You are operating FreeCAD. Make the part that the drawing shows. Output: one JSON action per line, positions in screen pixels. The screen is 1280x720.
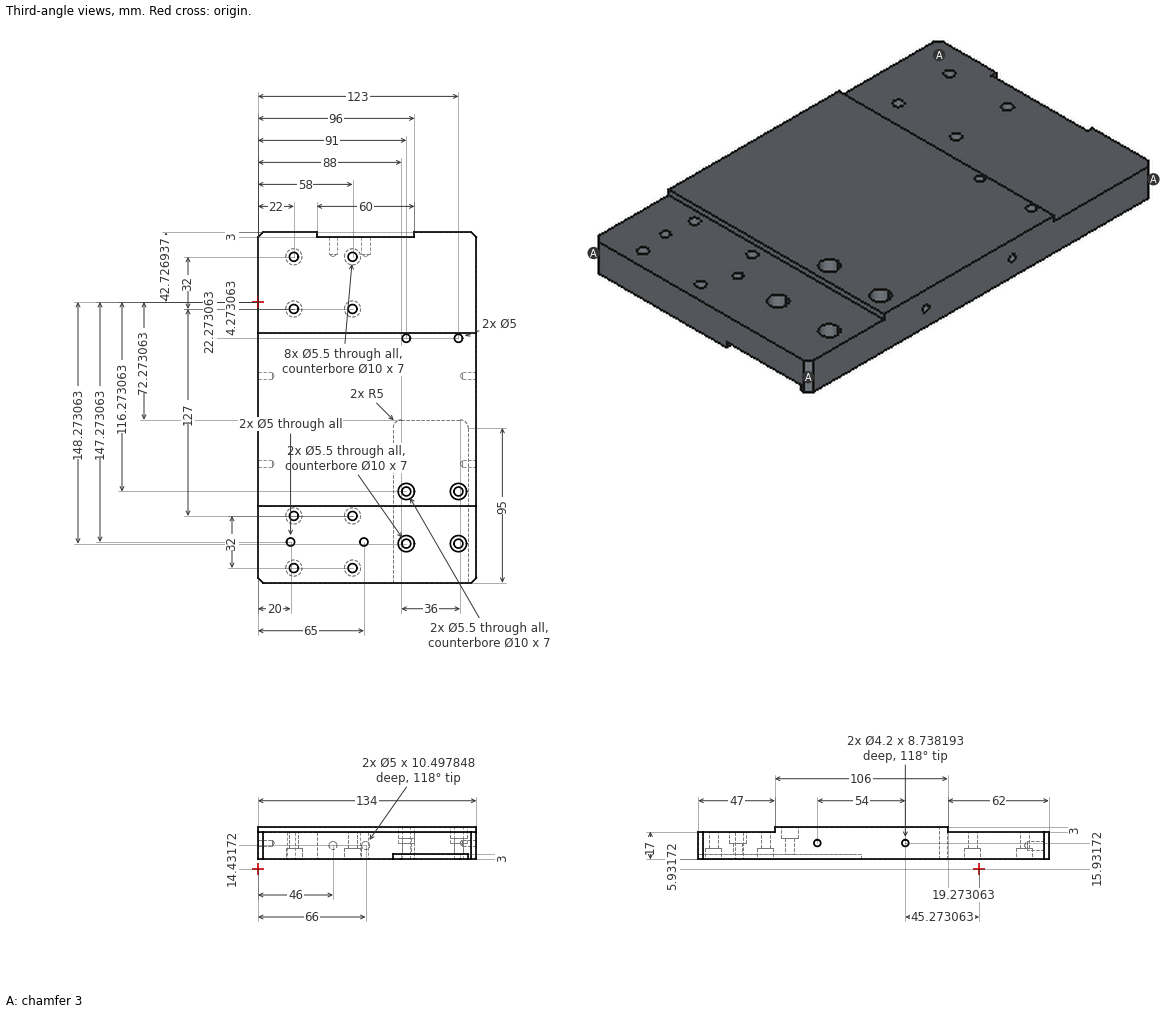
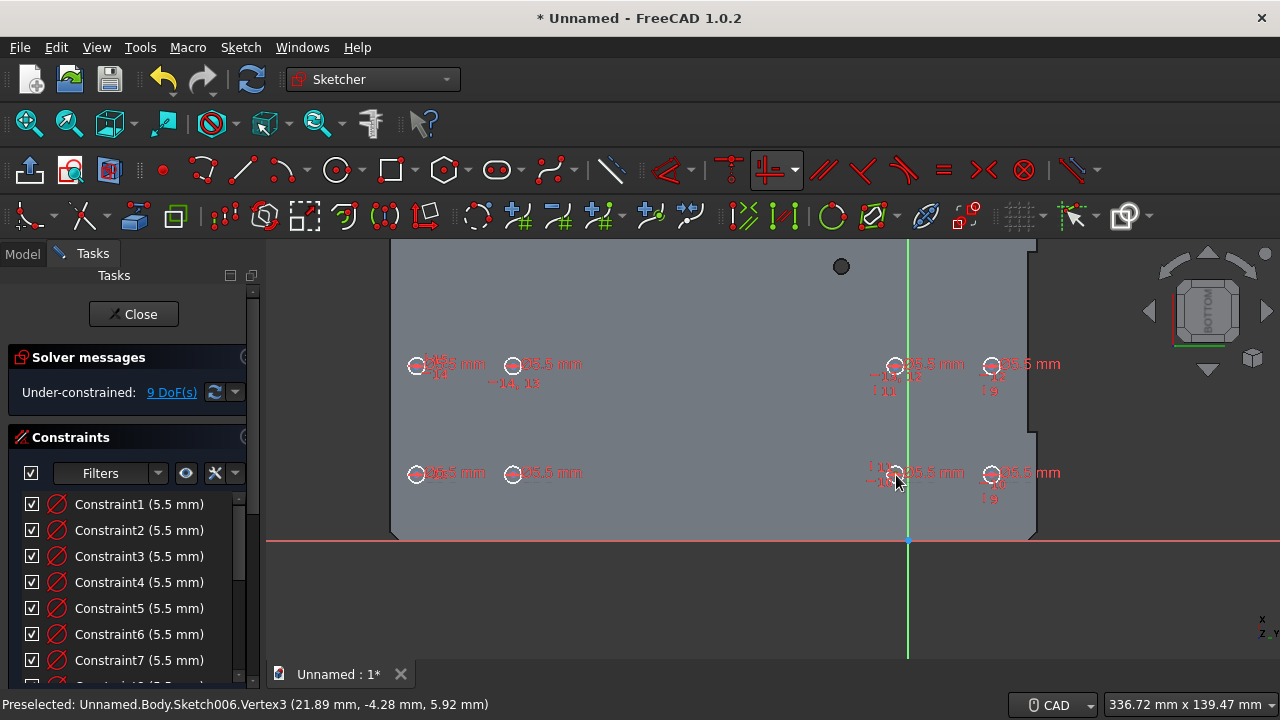
{"action": "left_click", "coordinate": [417, 475]}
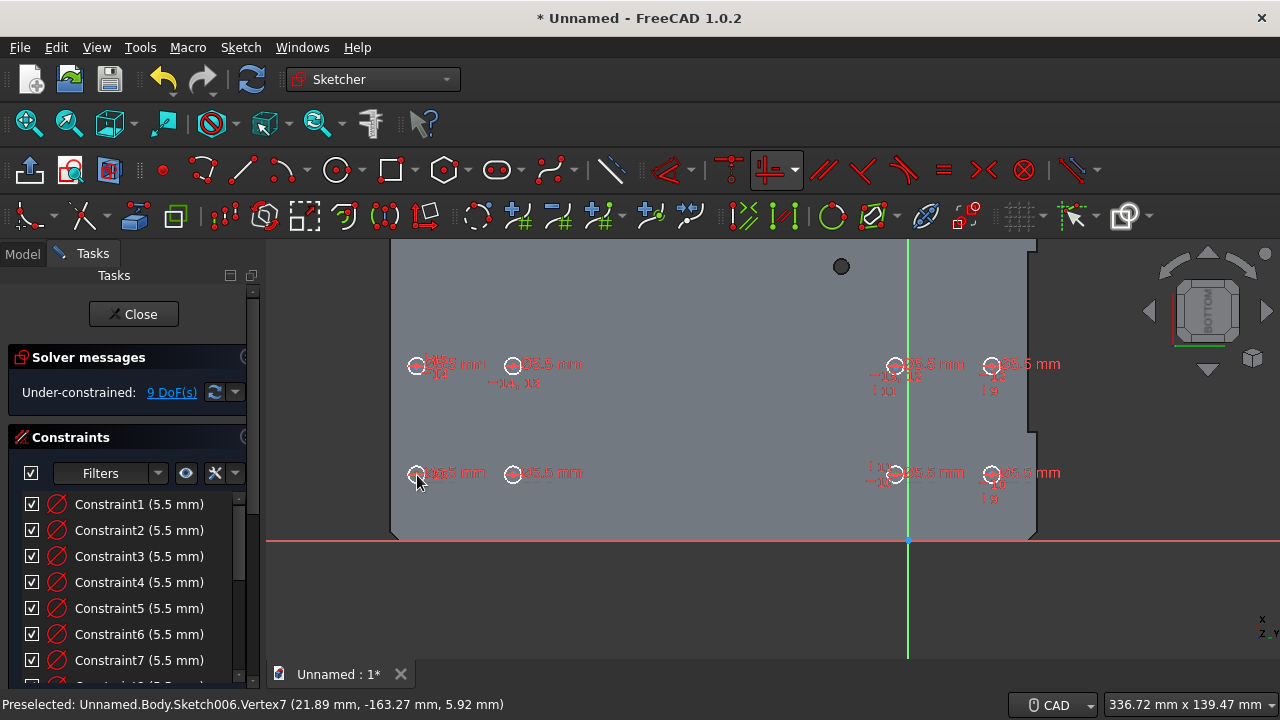
{"action": "key", "text": "h"}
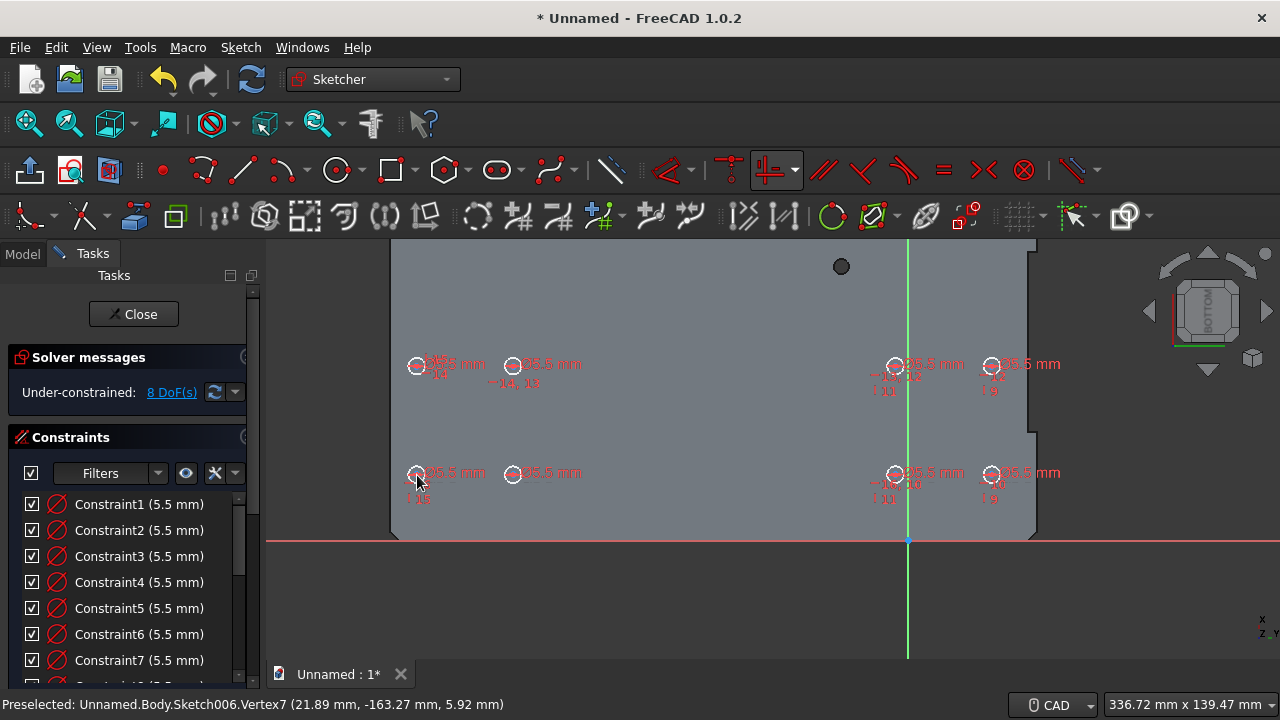
{"action": "left_click", "coordinate": [513, 366]}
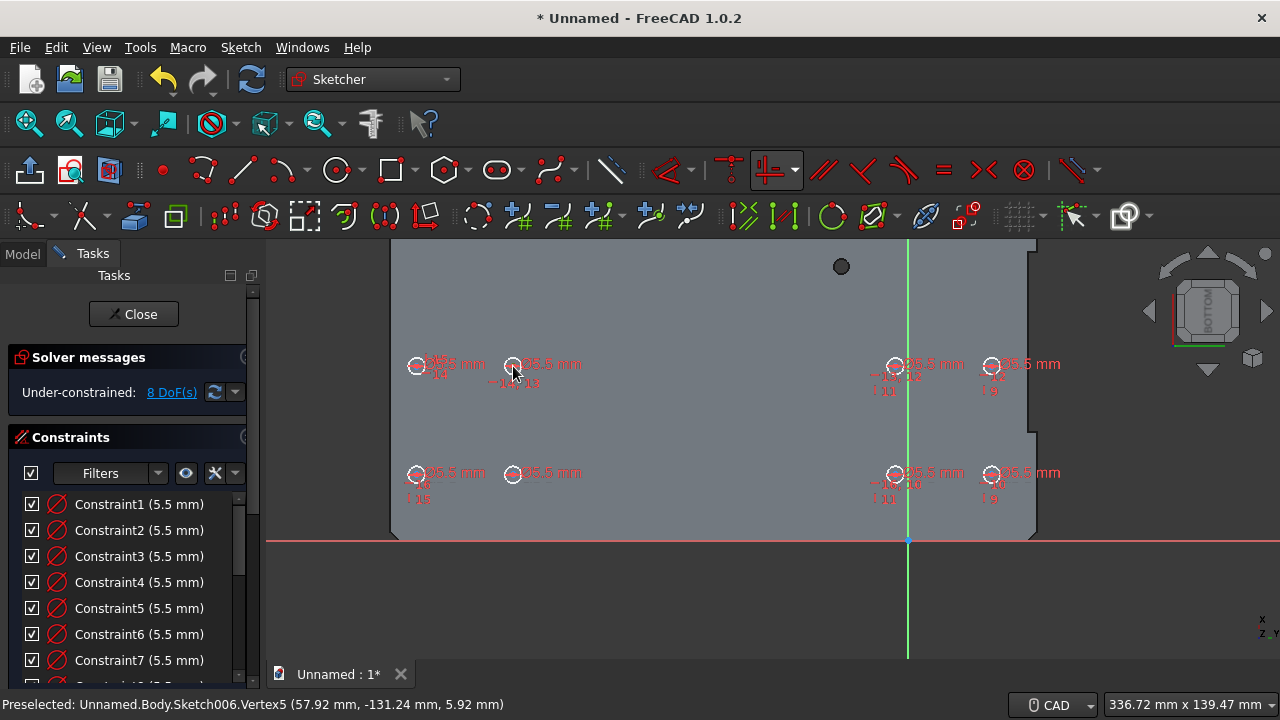
{"action": "left_click", "coordinate": [513, 475]}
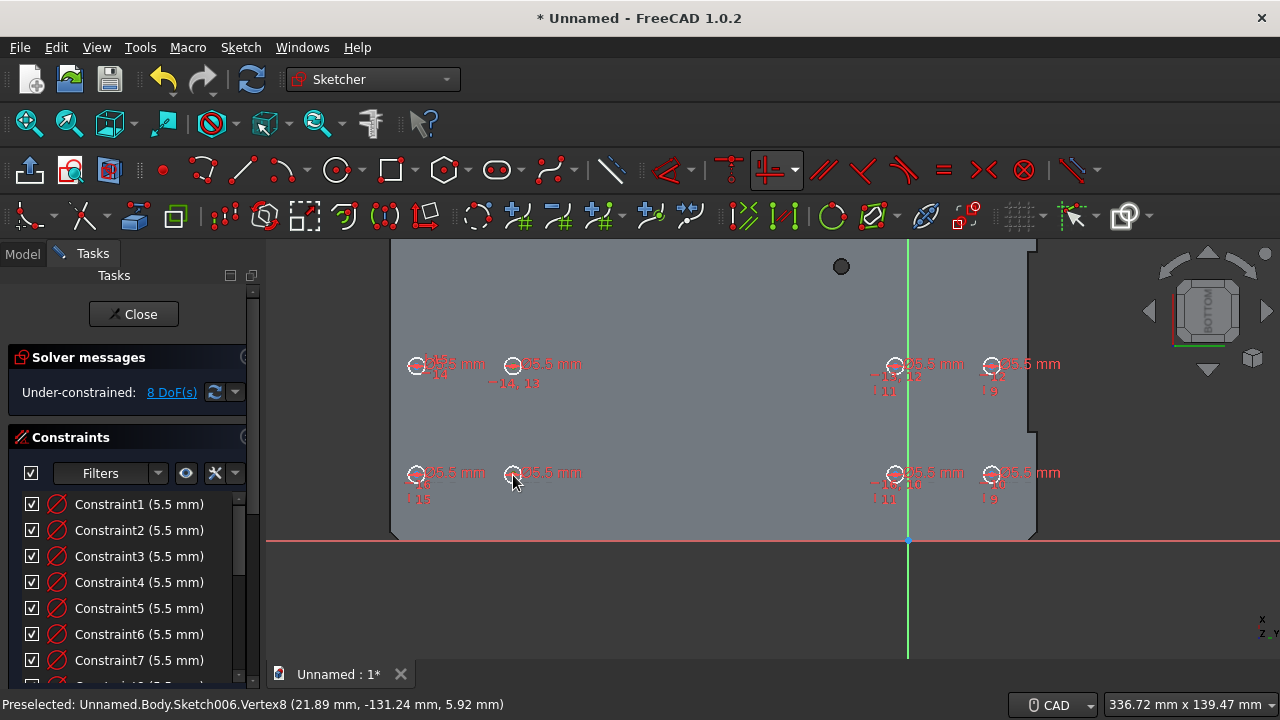
{"action": "left_click", "coordinate": [798, 170]}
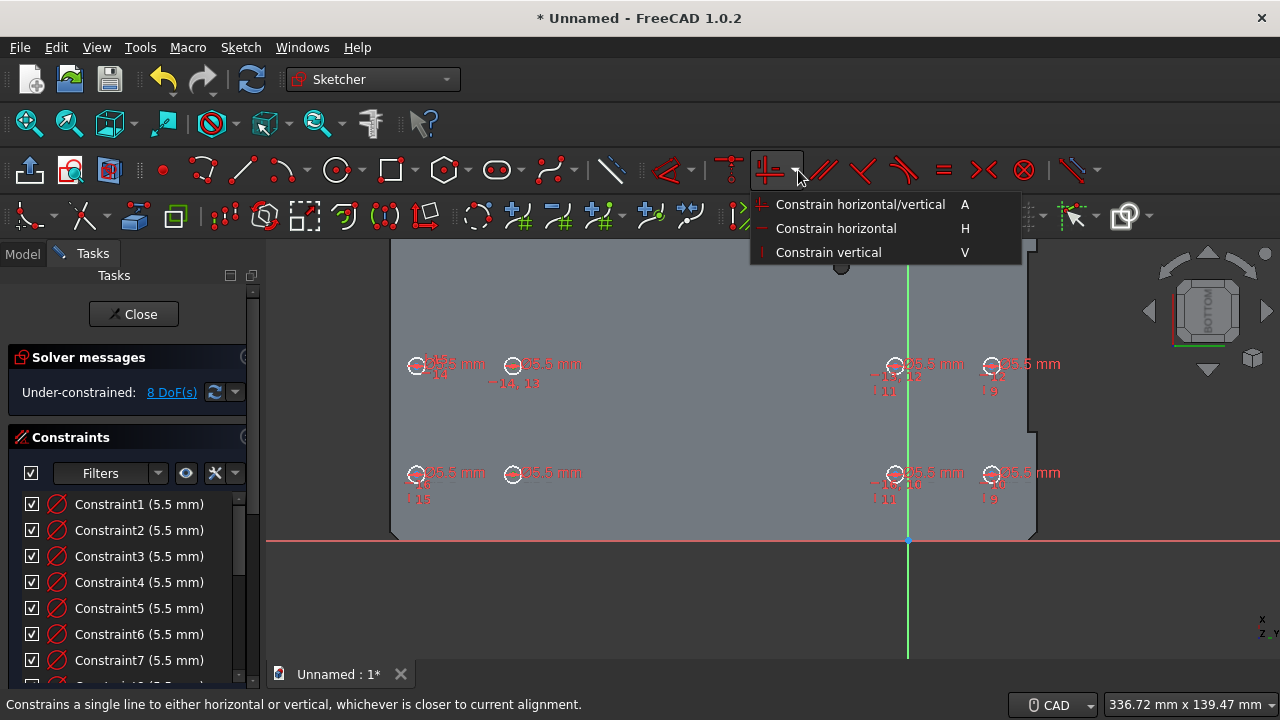
{"action": "left_click", "coordinate": [886, 252]}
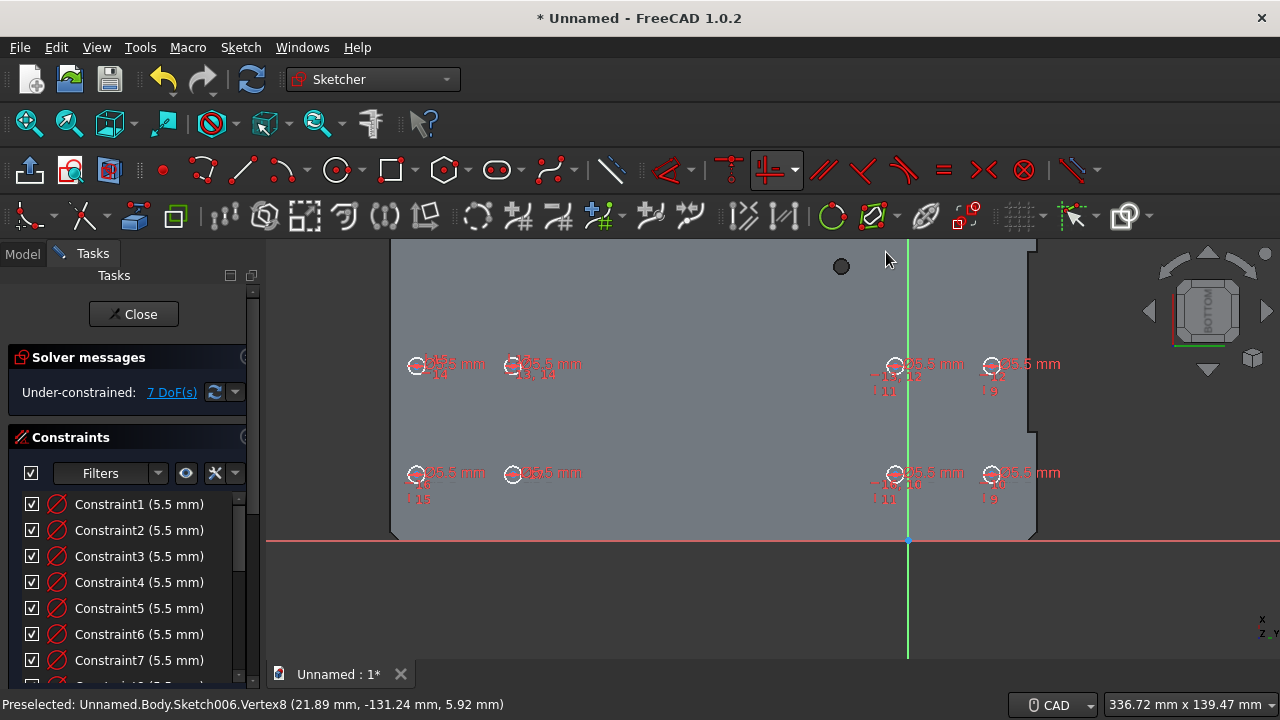
{"action": "left_click", "coordinate": [417, 475]}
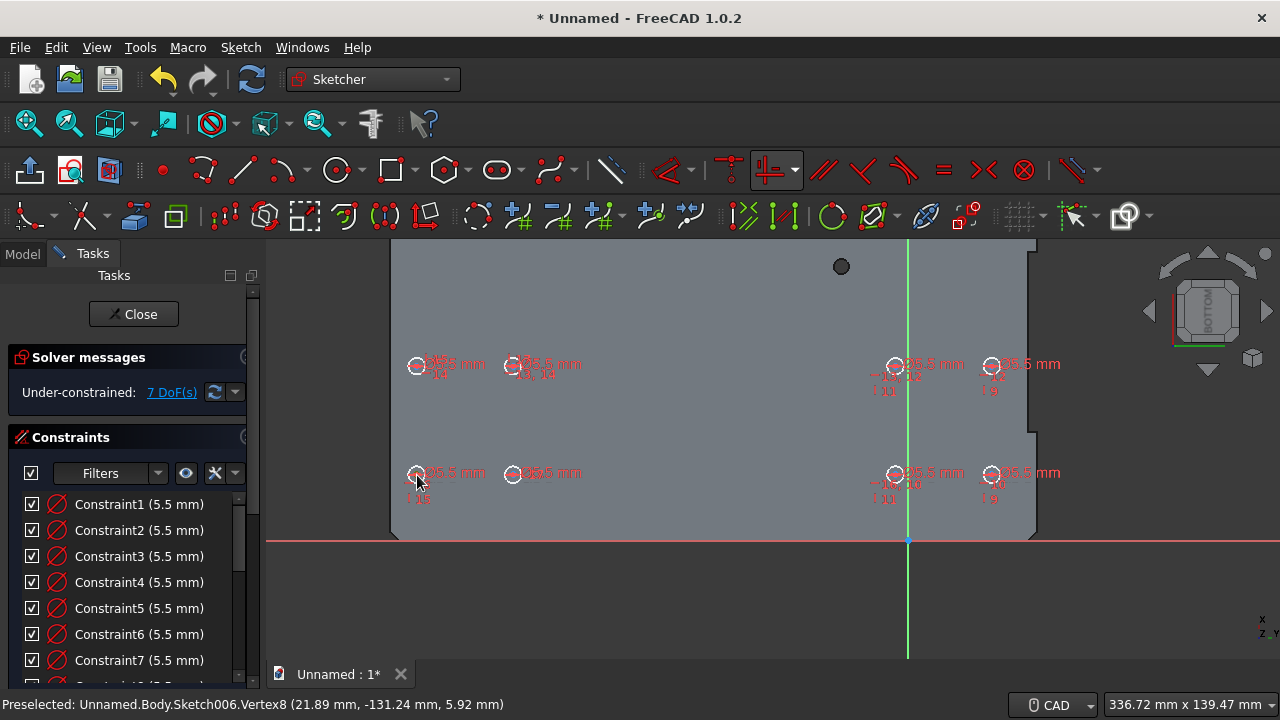
{"action": "left_click", "coordinate": [513, 475]}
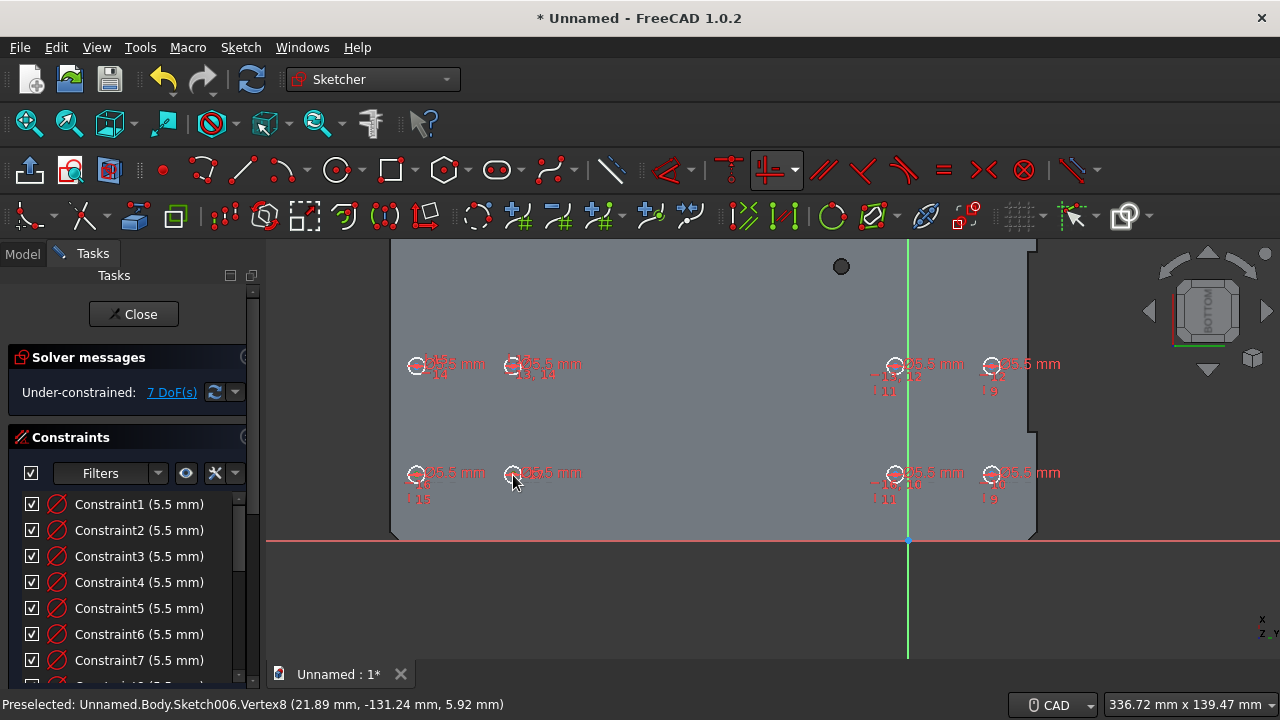
{"action": "left_click", "coordinate": [798, 170]}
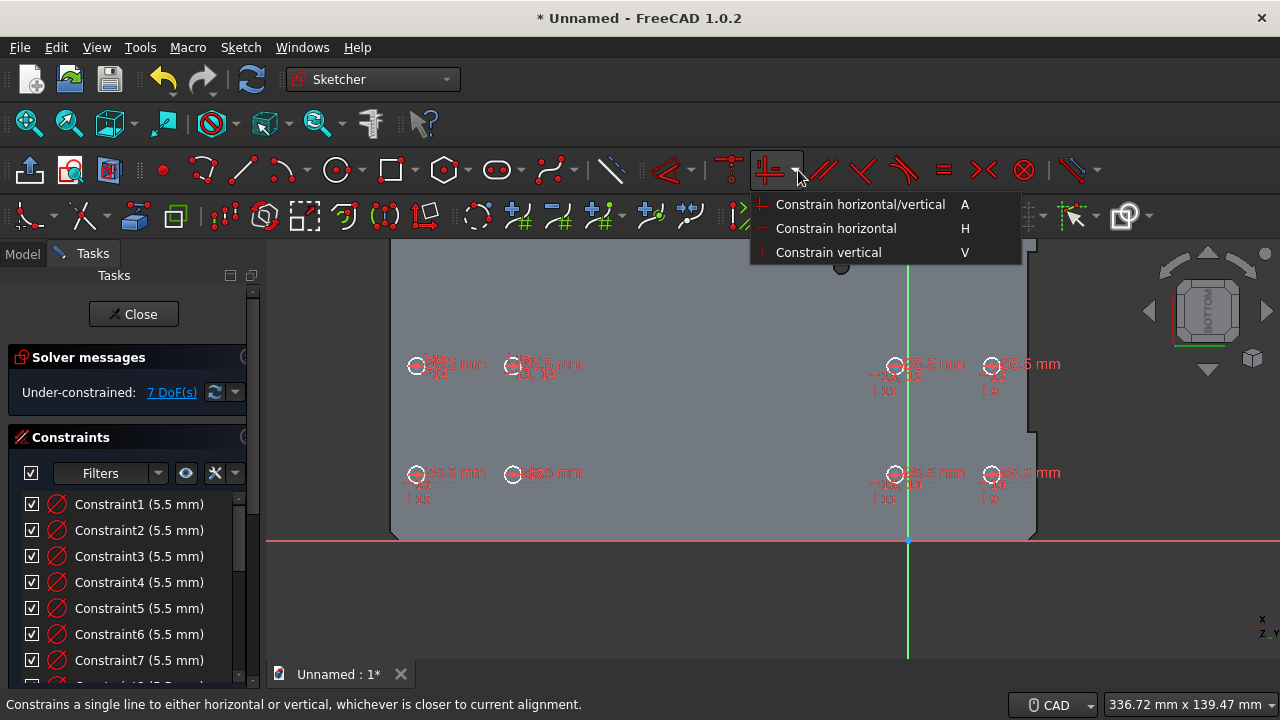
{"action": "left_click", "coordinate": [886, 228]}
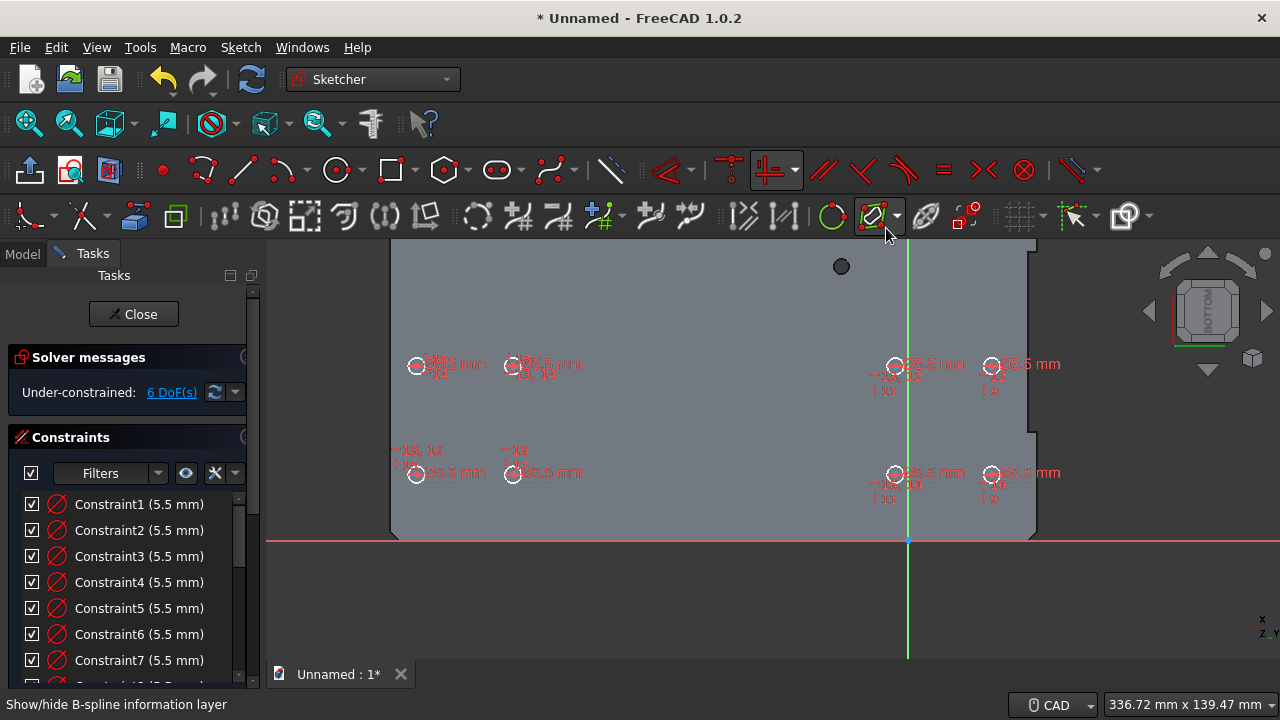
{"action": "left_click", "coordinate": [666, 170]}